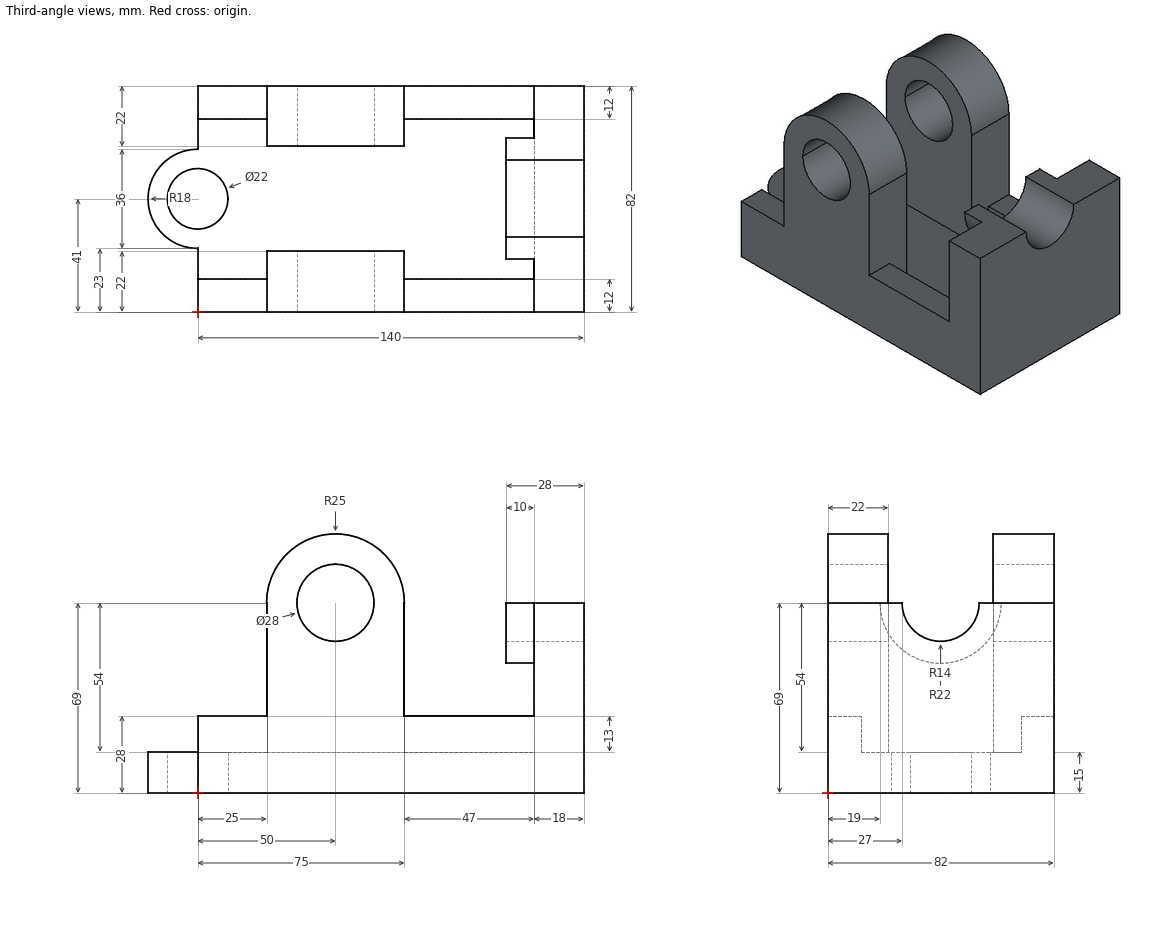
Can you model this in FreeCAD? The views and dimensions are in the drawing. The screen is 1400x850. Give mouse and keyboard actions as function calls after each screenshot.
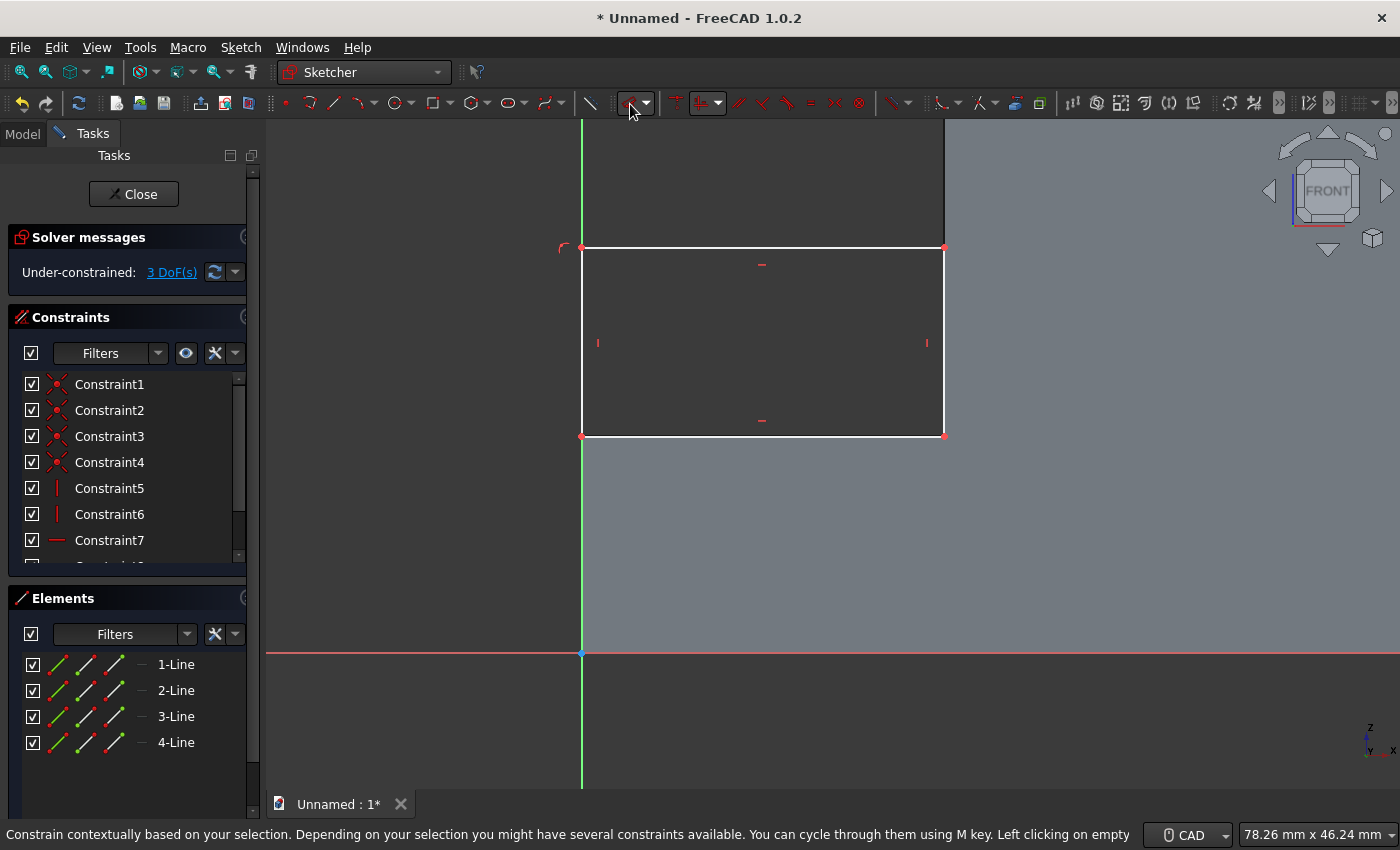
click(582, 305)
click(548, 343)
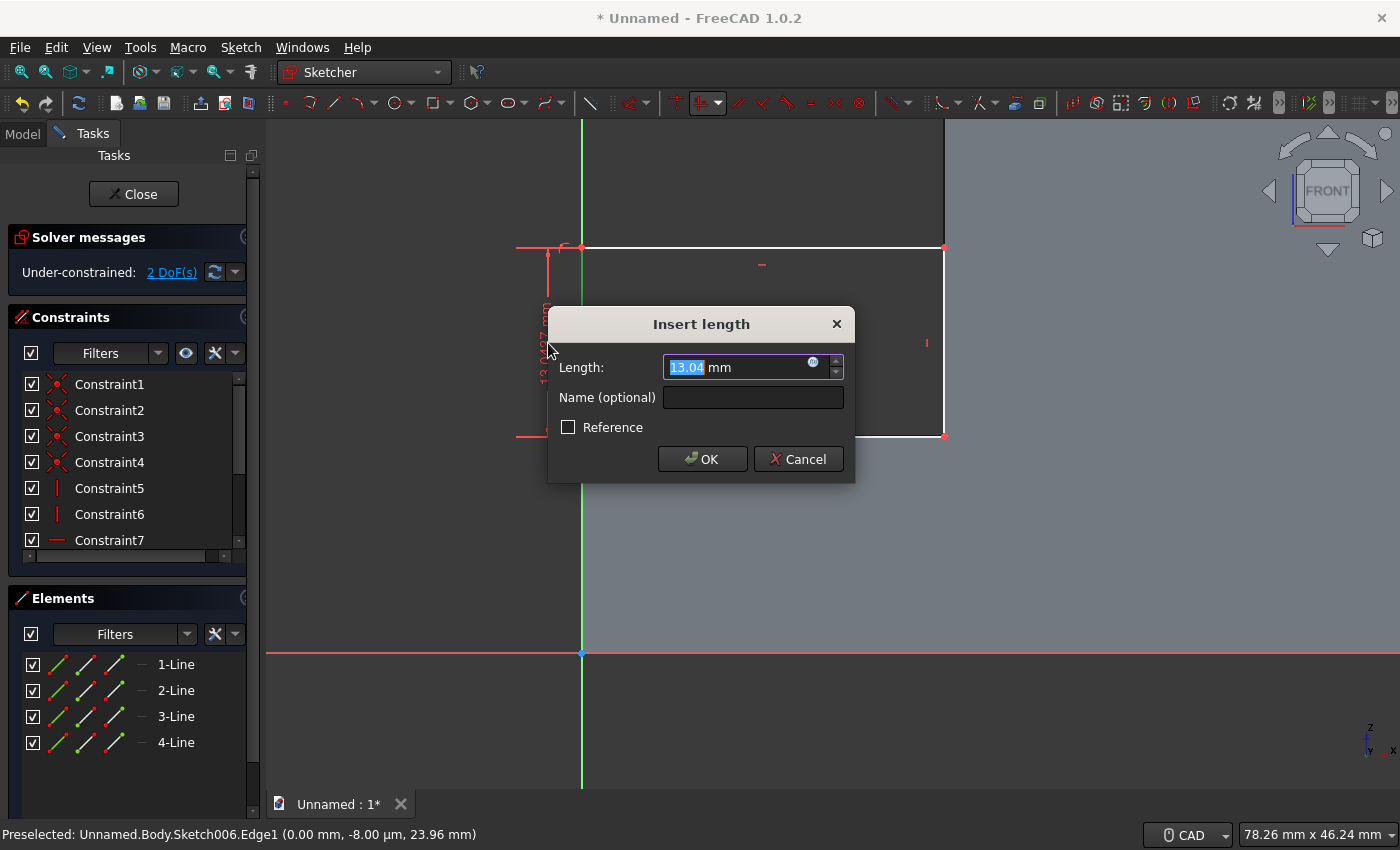
text(13)
key(Return)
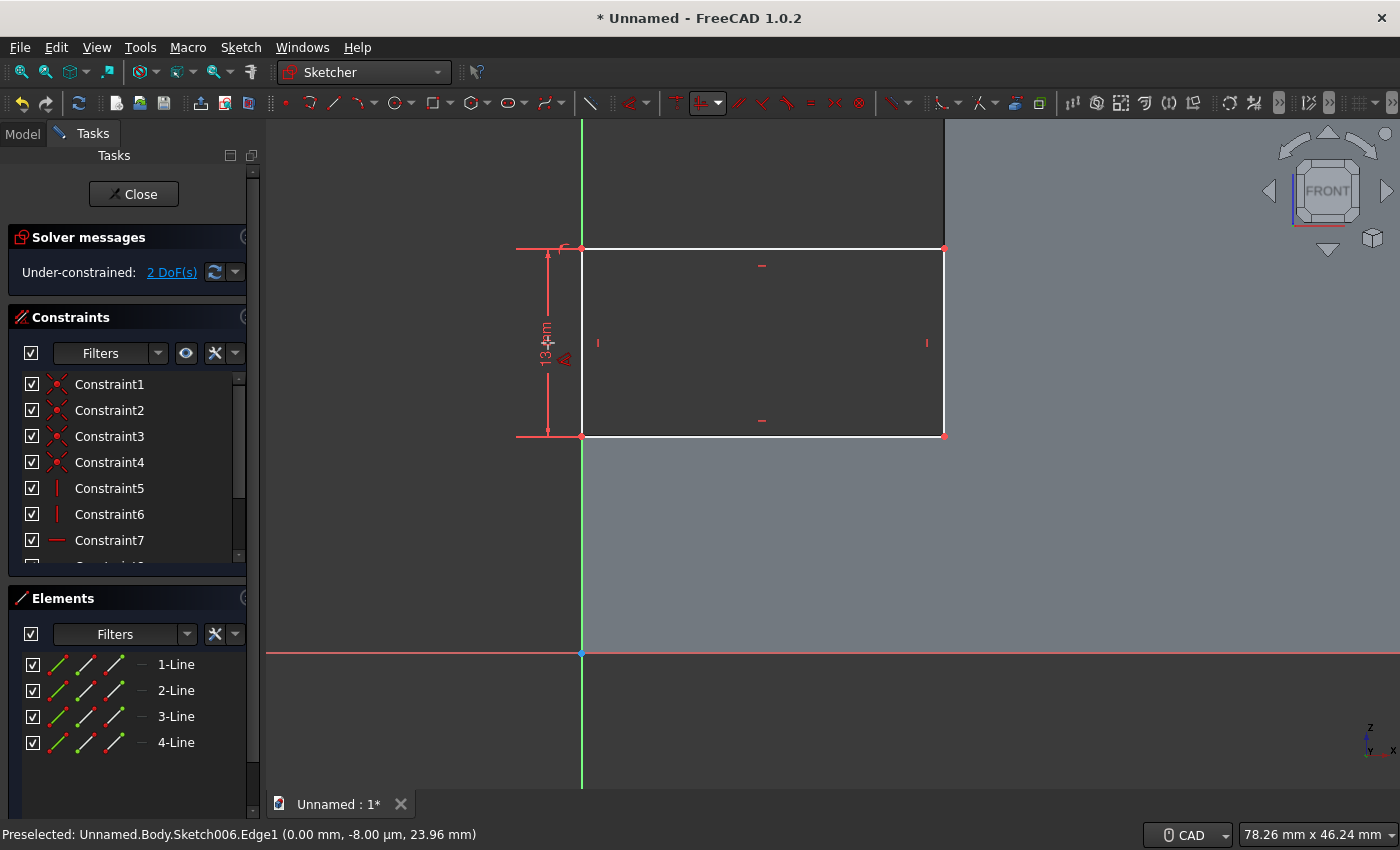
click(690, 437)
click(763, 403)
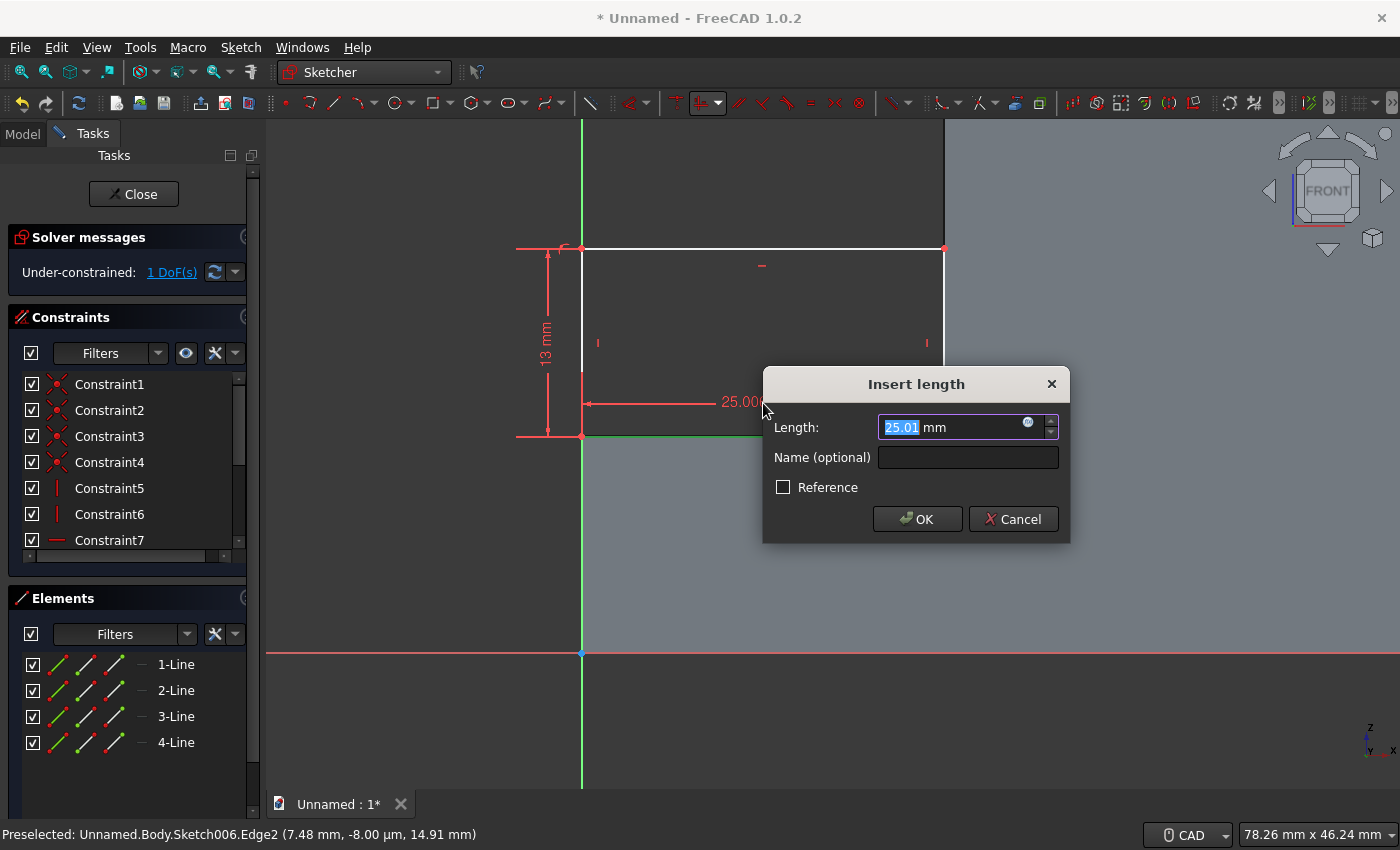
text(25)
key(Return)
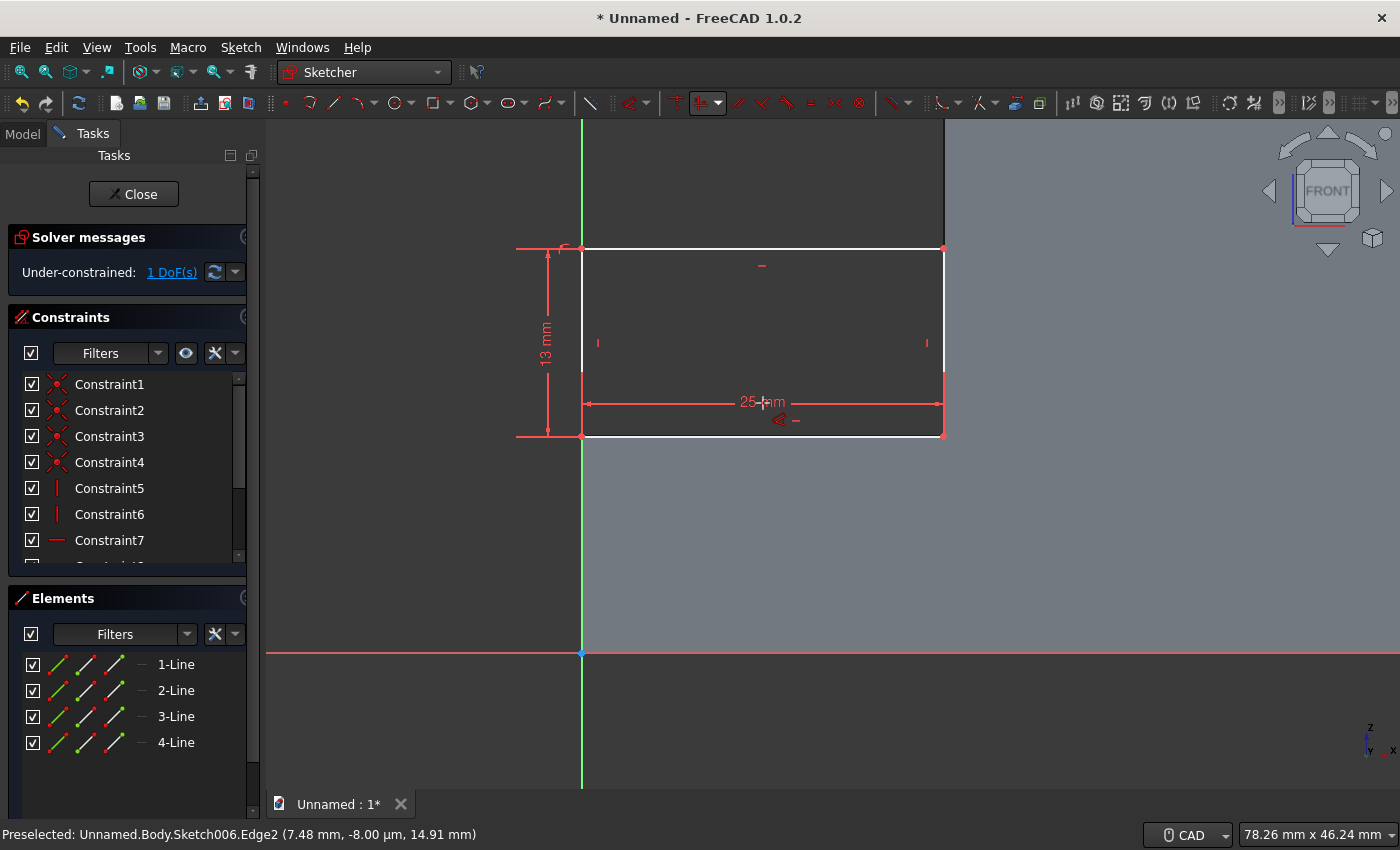
click(582, 249)
click(548, 451)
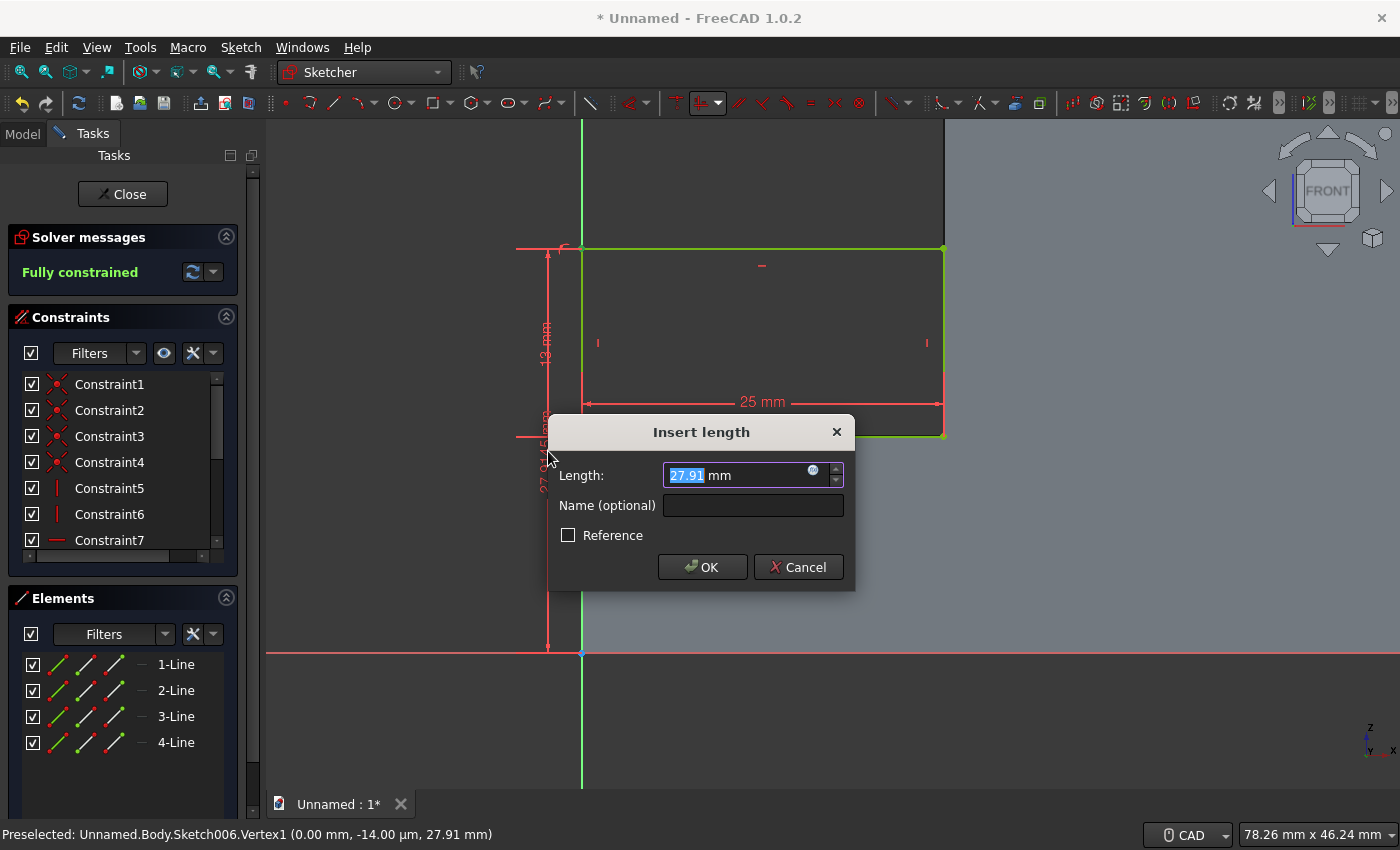
text(28)
key(Return)
key(Escape)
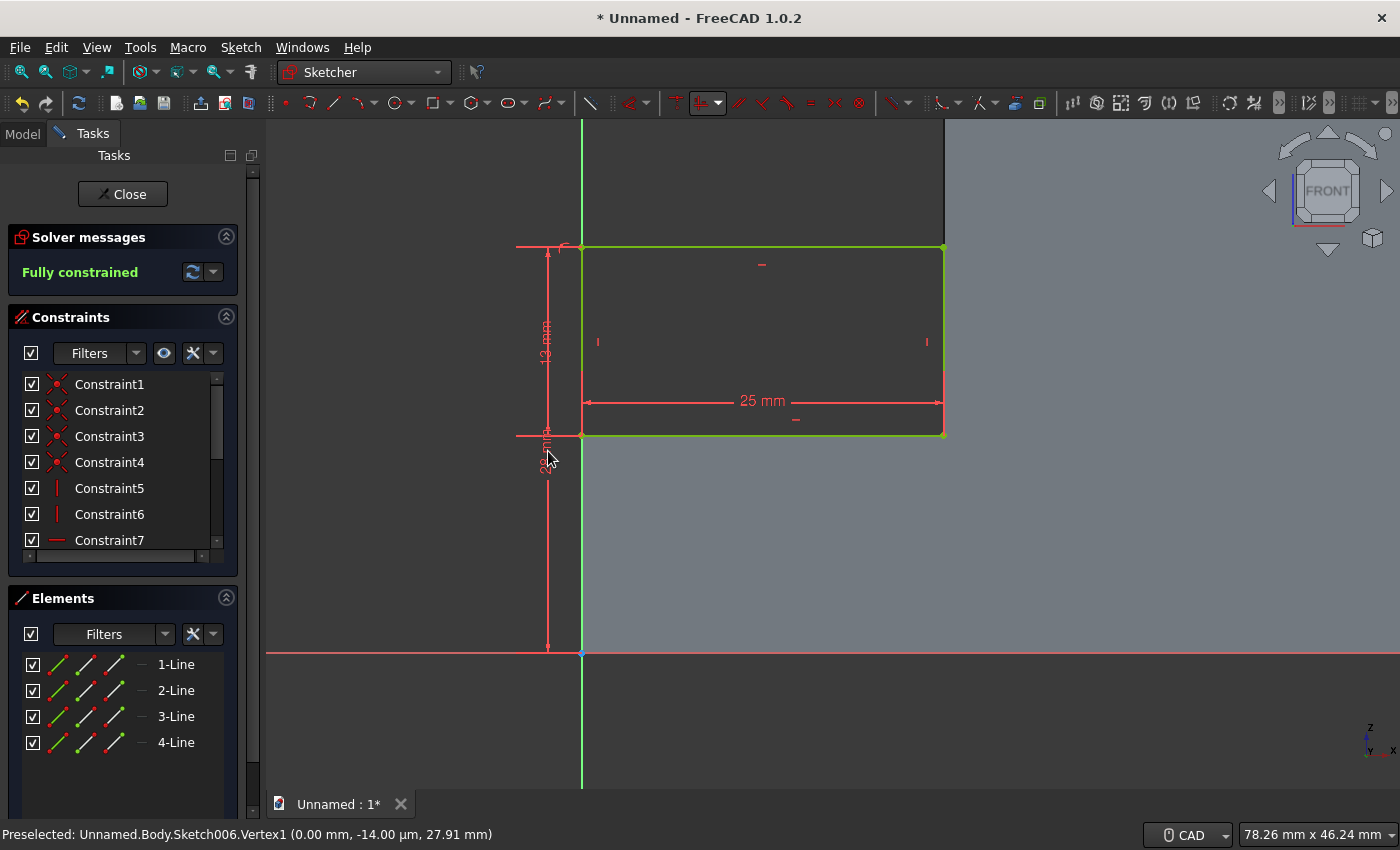
click(123, 194)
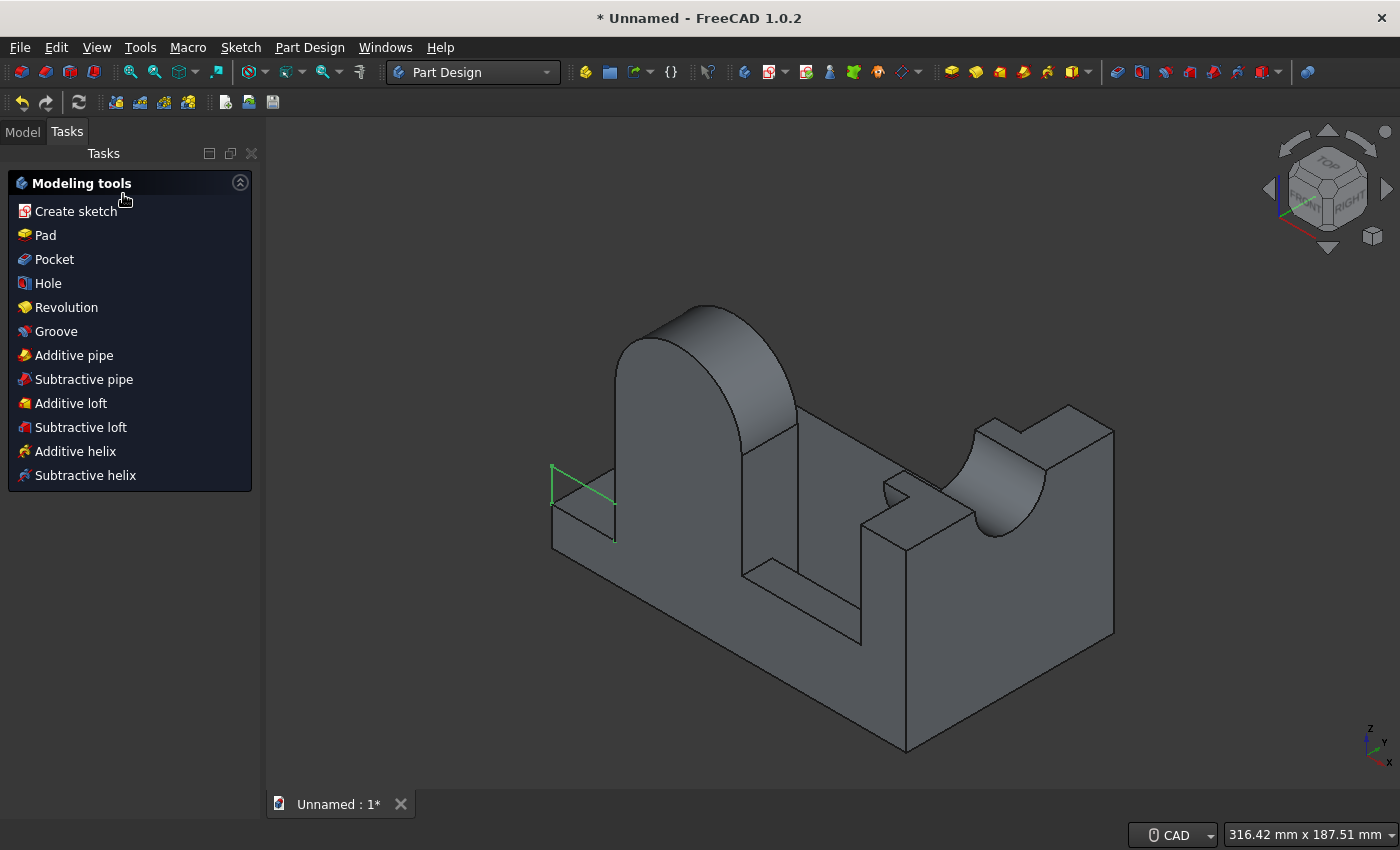
click(952, 72)